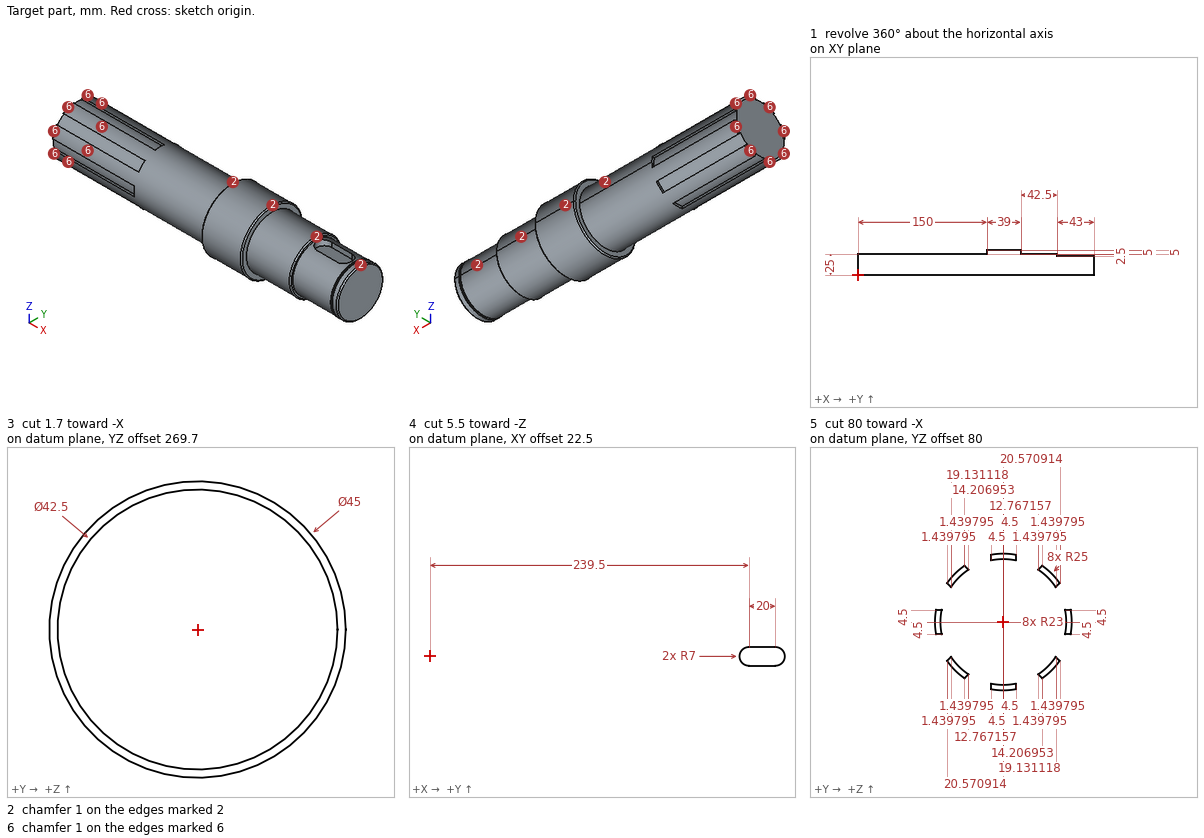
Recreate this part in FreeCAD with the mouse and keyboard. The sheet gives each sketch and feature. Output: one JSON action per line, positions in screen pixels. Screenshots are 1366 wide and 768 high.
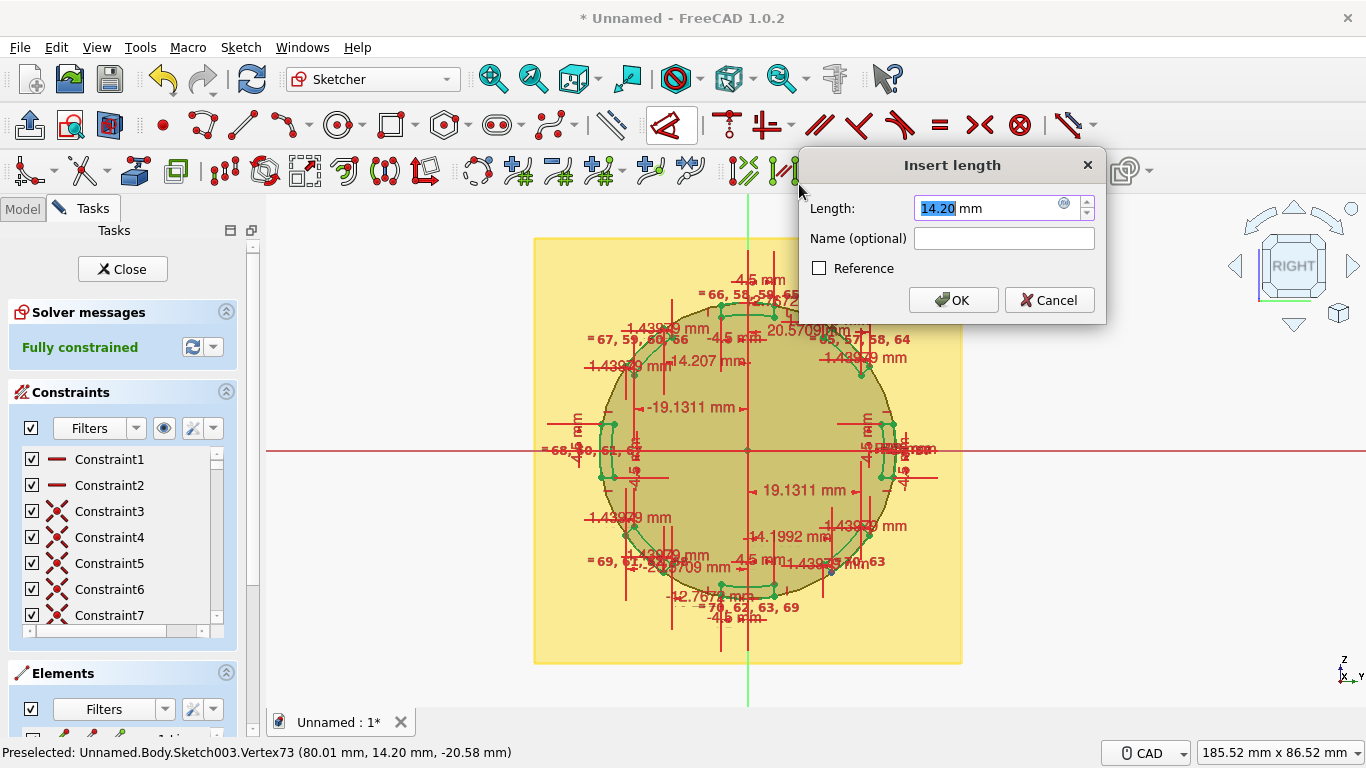
{"action": "type", "text": "14.206953"}
{"action": "key", "text": "Return"}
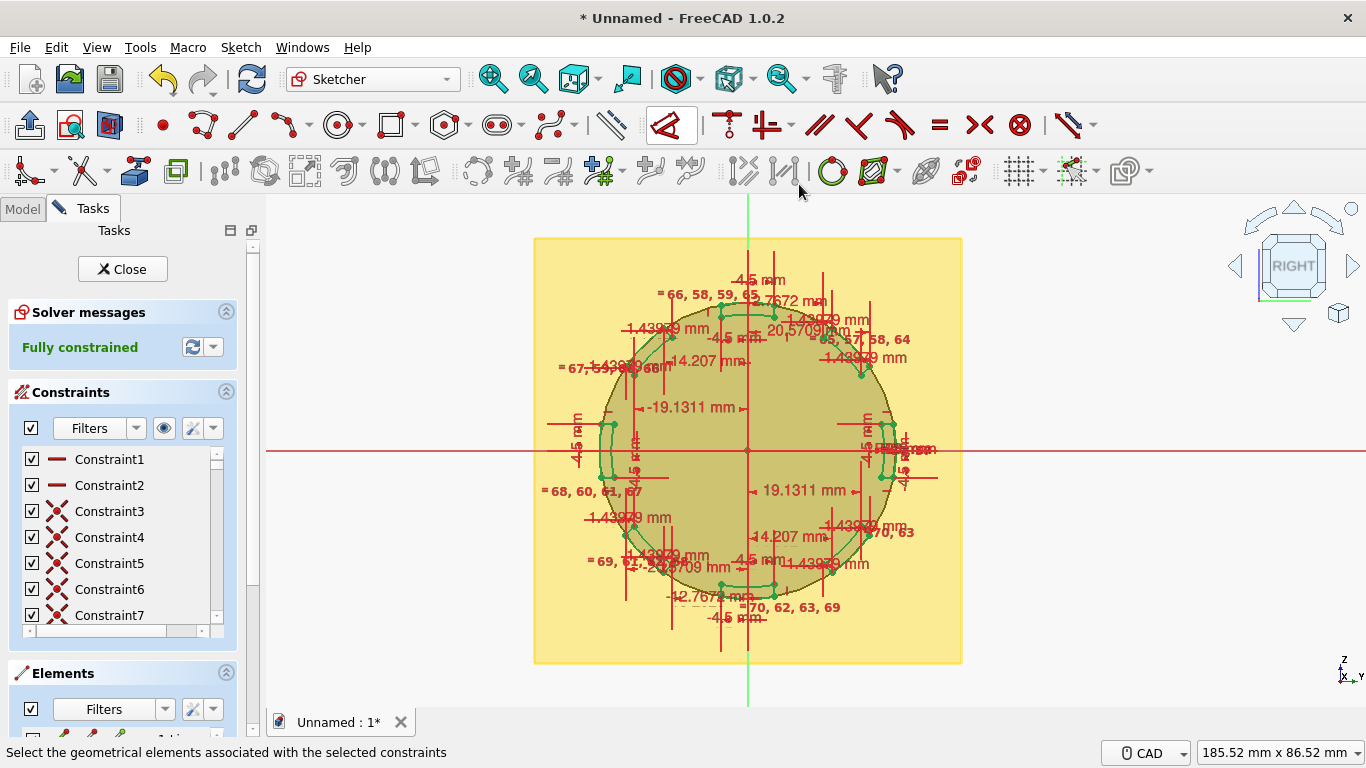
{"action": "left_click", "coordinate": [123, 269]}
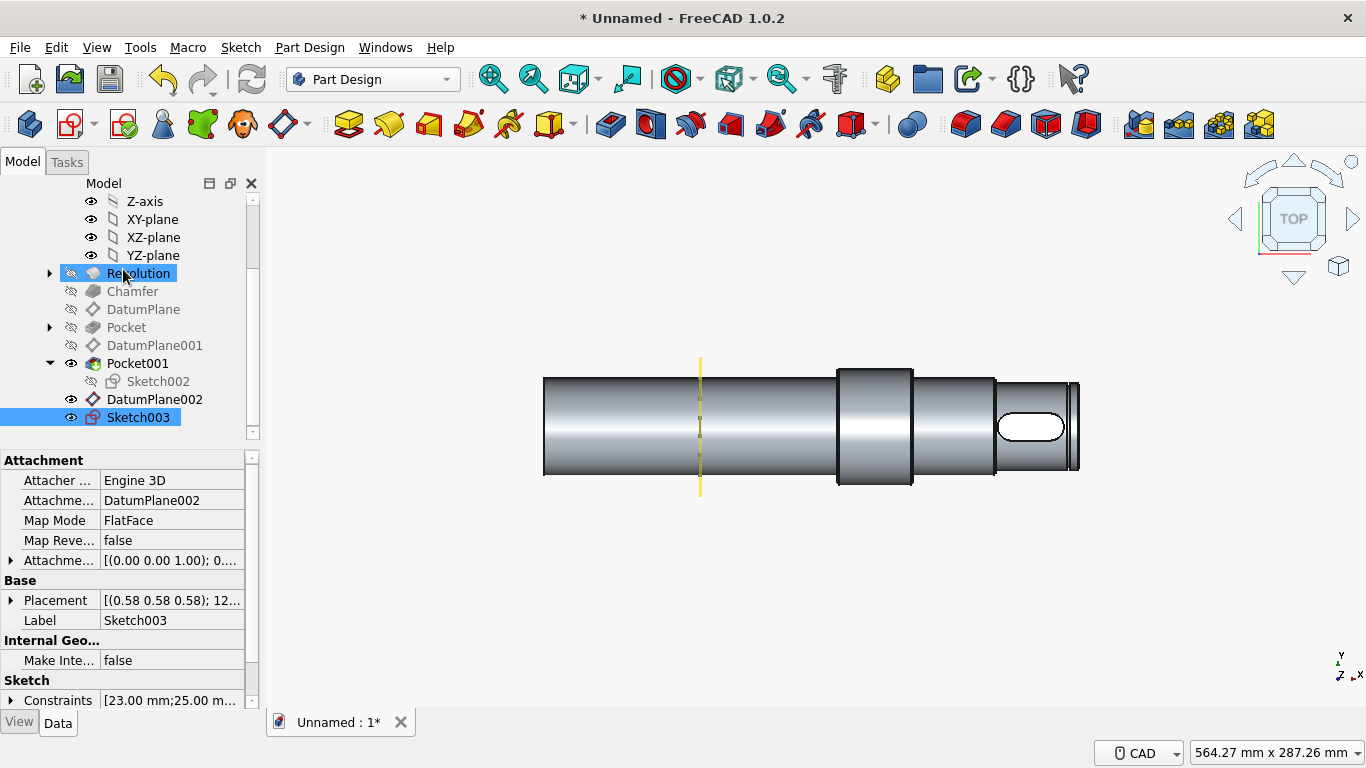
{"action": "left_click", "coordinate": [612, 124]}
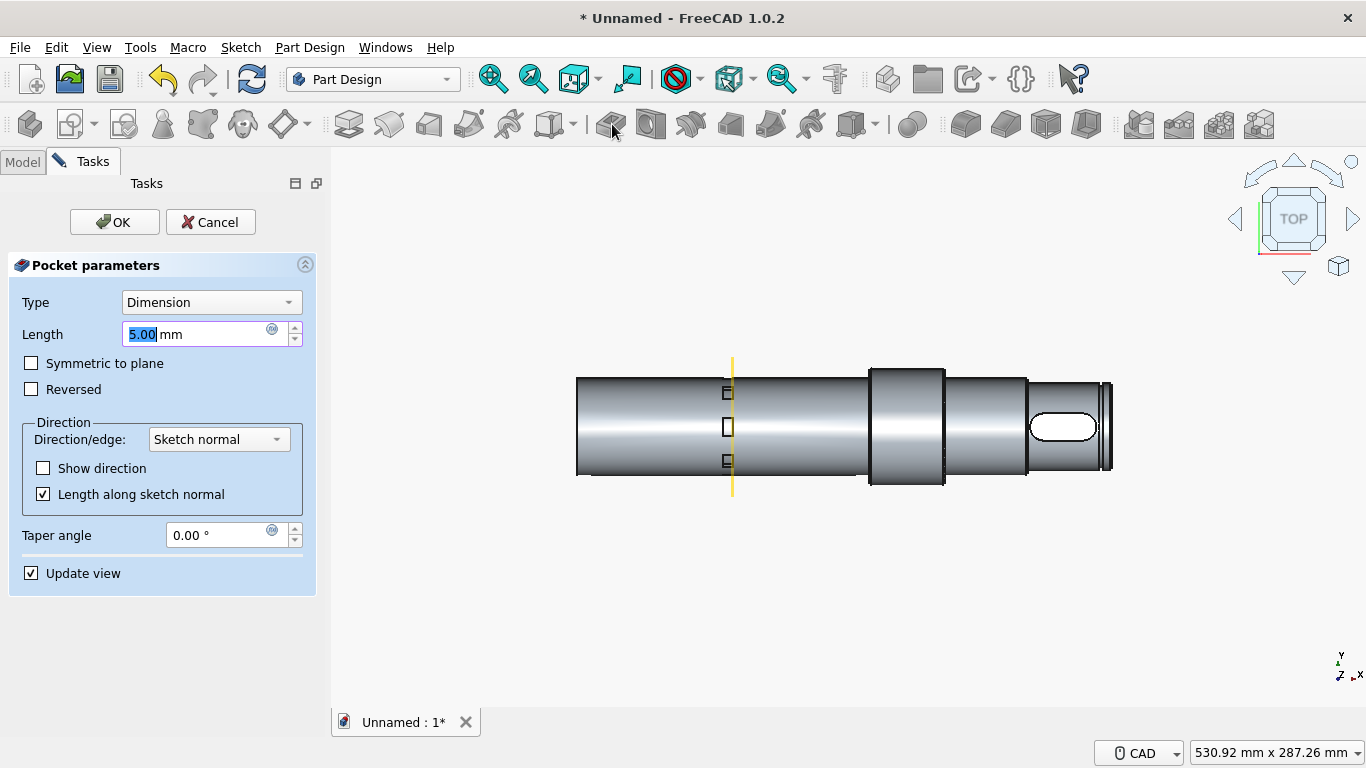
{"action": "type", "text": "80"}
{"action": "key", "text": "Tab"}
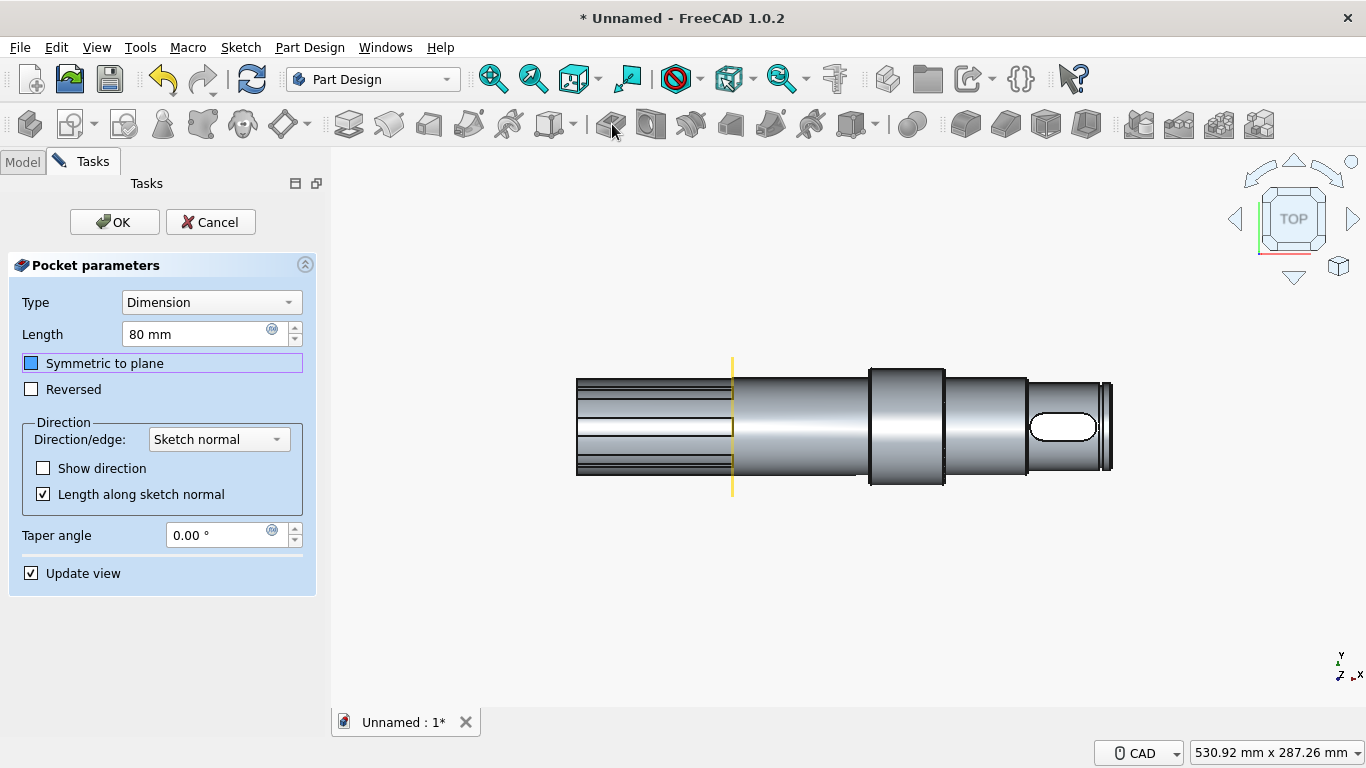
{"action": "left_click", "coordinate": [115, 222]}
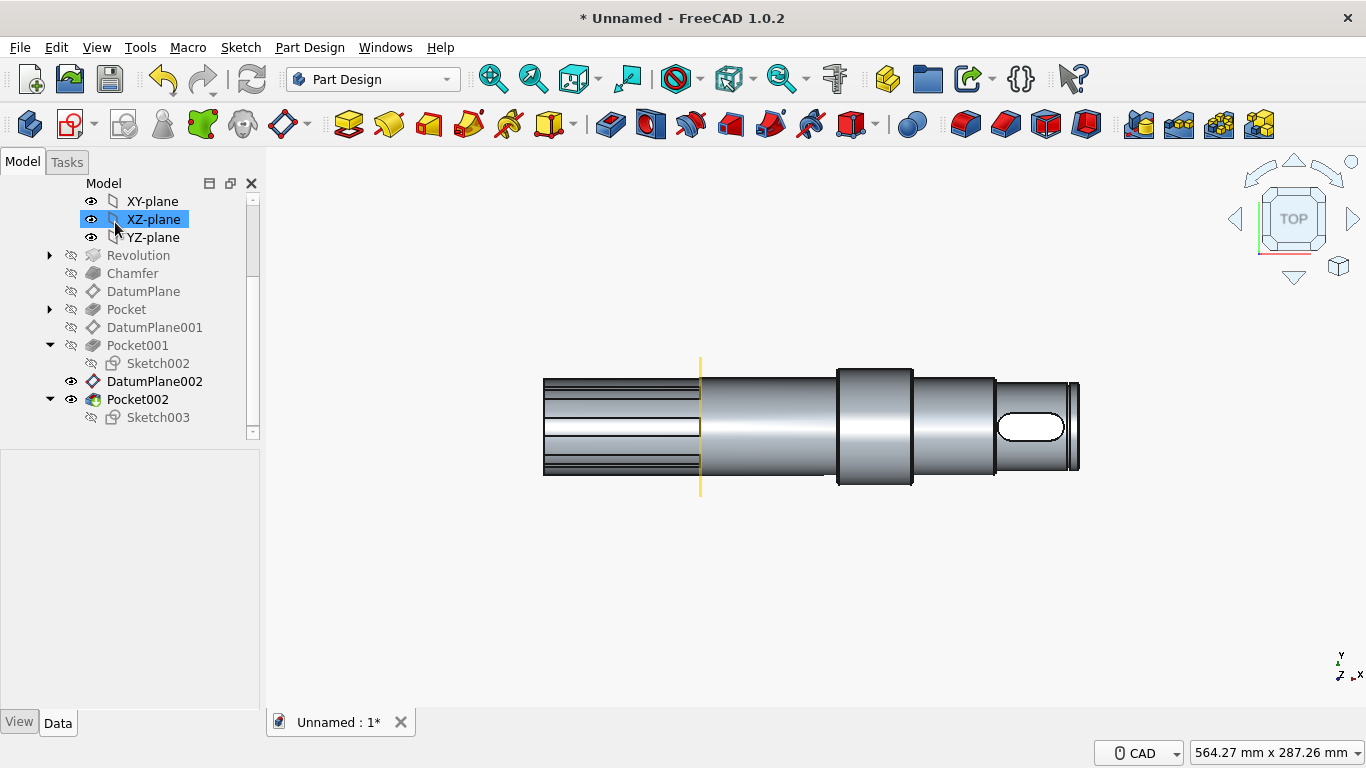
{"action": "left_click", "coordinate": [116, 381]}
{"action": "key", "text": "space"}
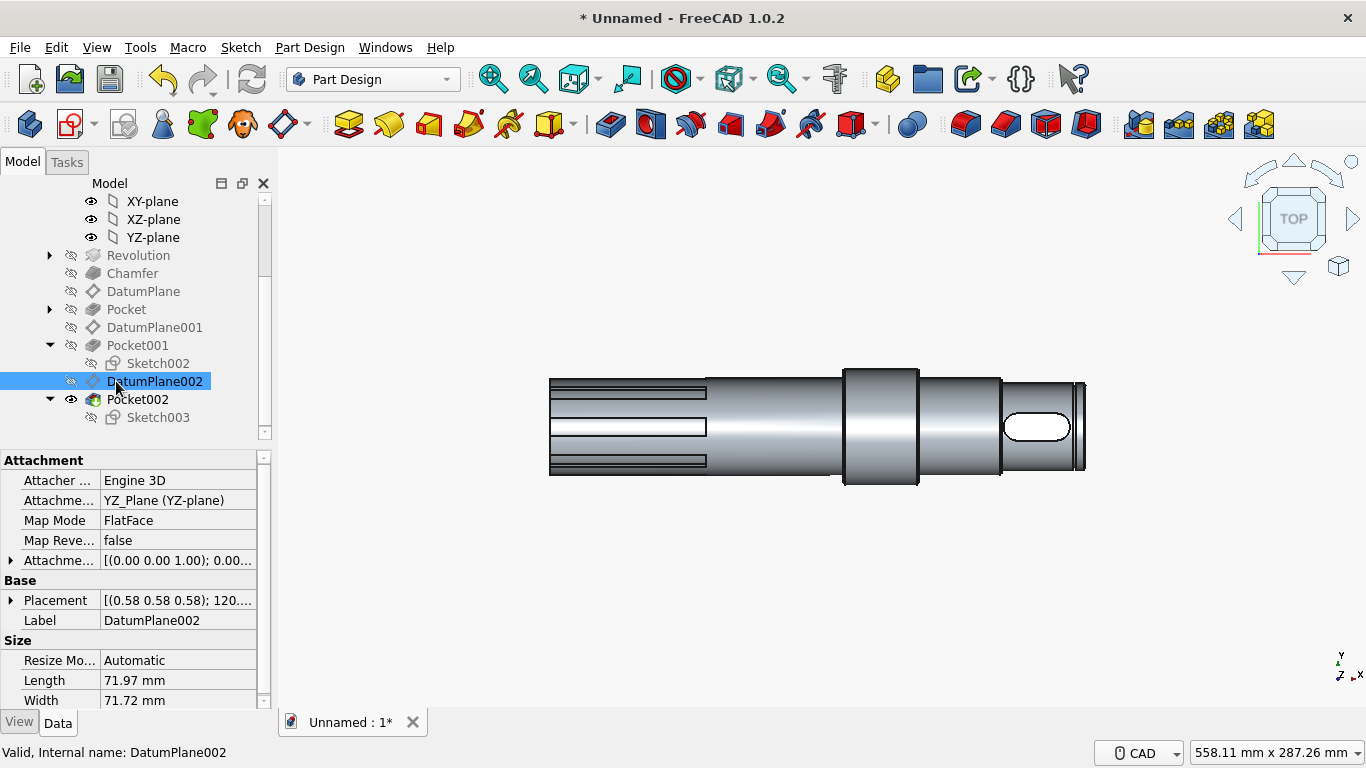
{"action": "left_click", "coordinate": [550, 379]}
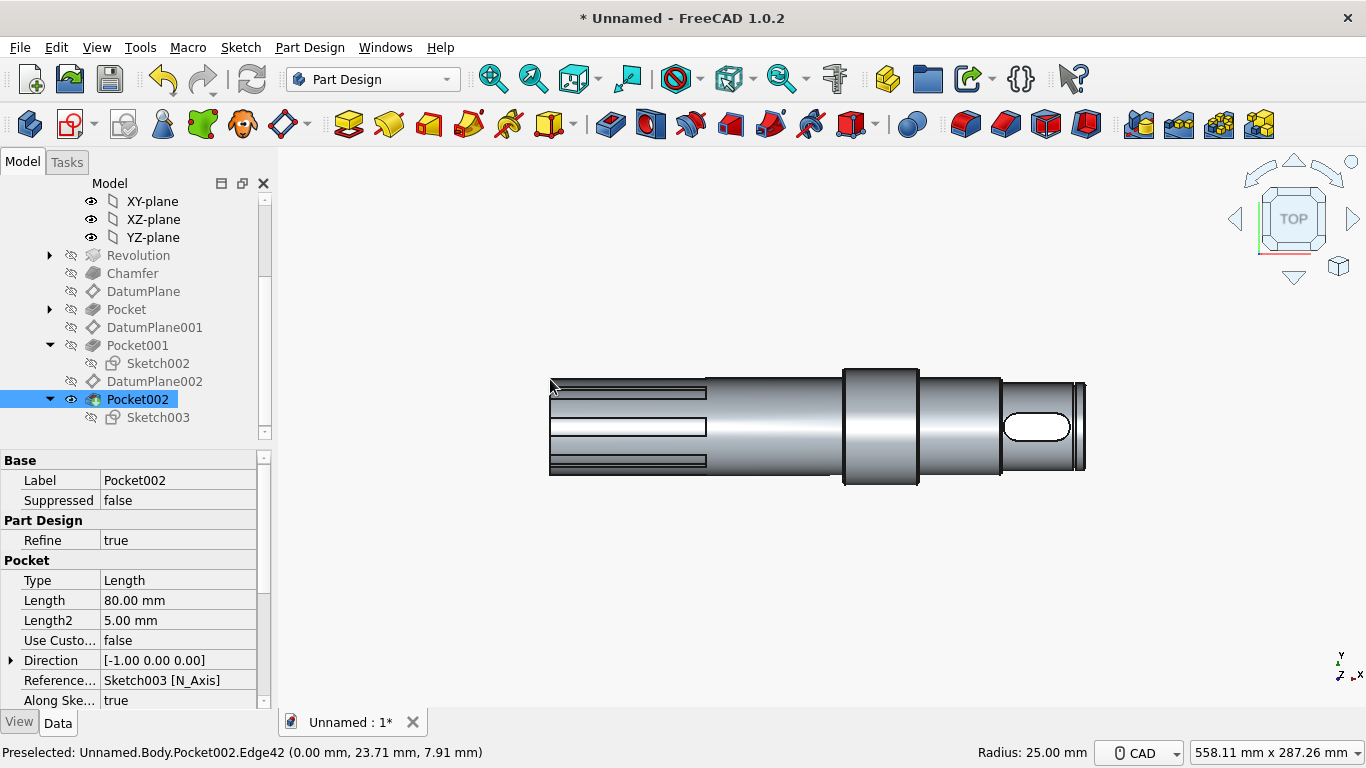
{"action": "left_click", "coordinate": [550, 407], "text": "ctrl"}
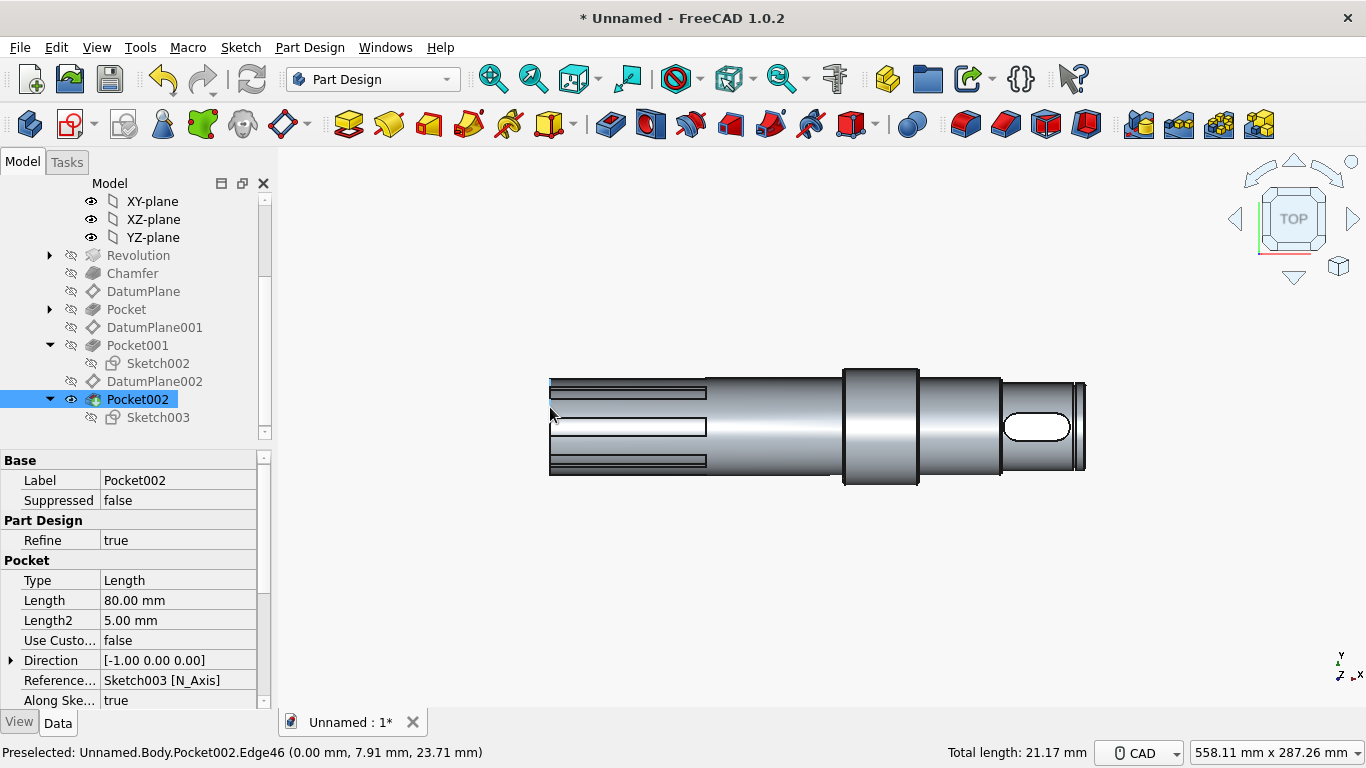
{"action": "left_click", "coordinate": [550, 445], "text": "ctrl"}